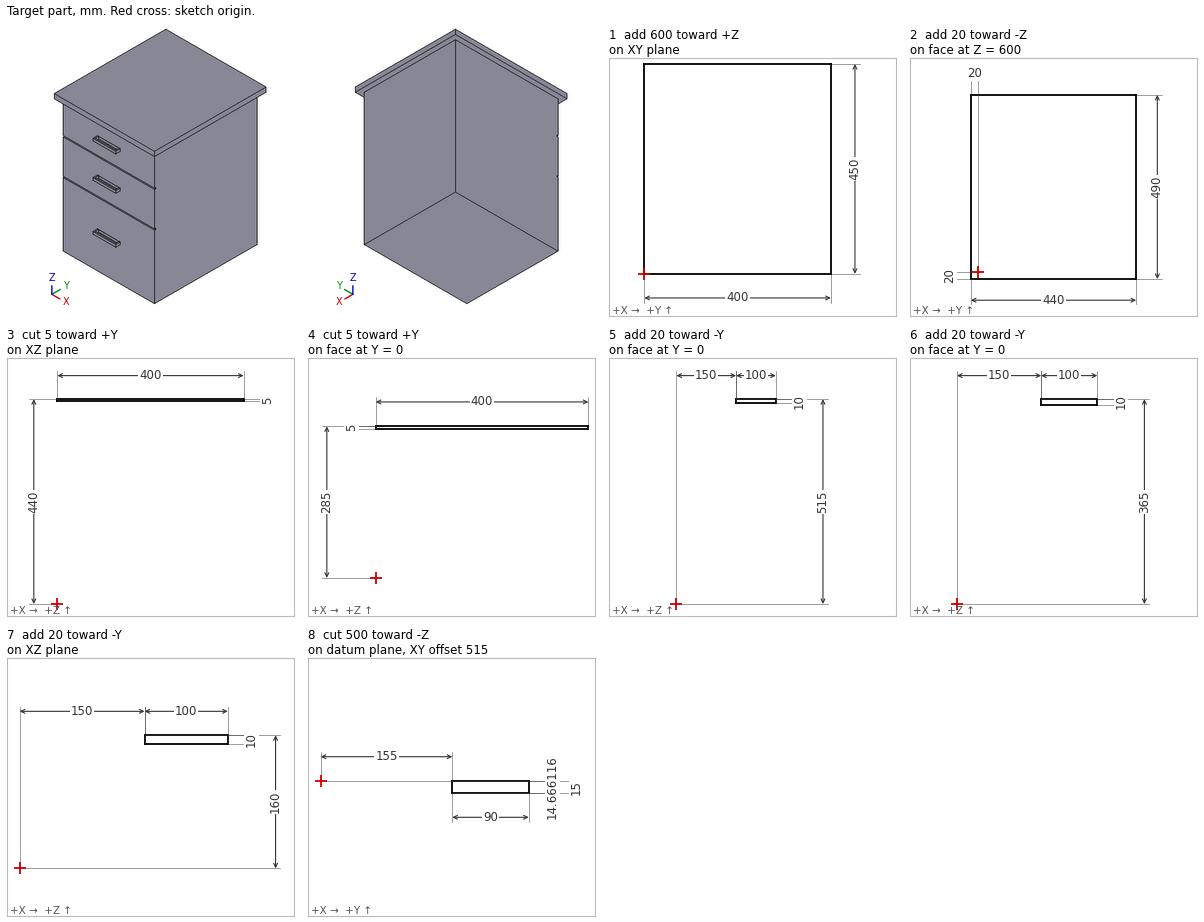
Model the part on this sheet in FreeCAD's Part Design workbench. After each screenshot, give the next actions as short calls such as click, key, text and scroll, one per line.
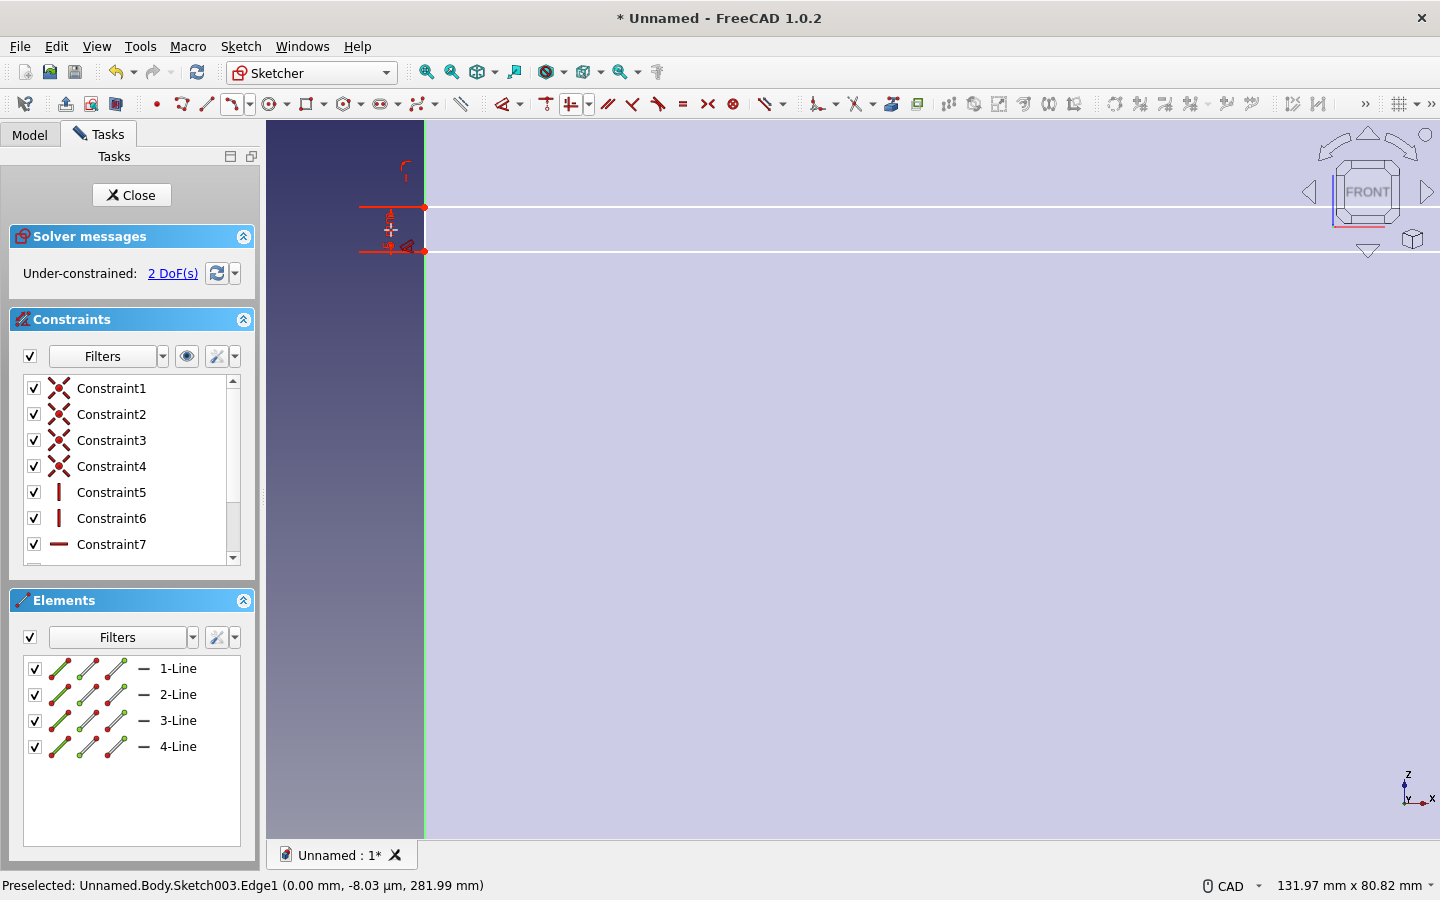
scroll(425, 228, down, 8)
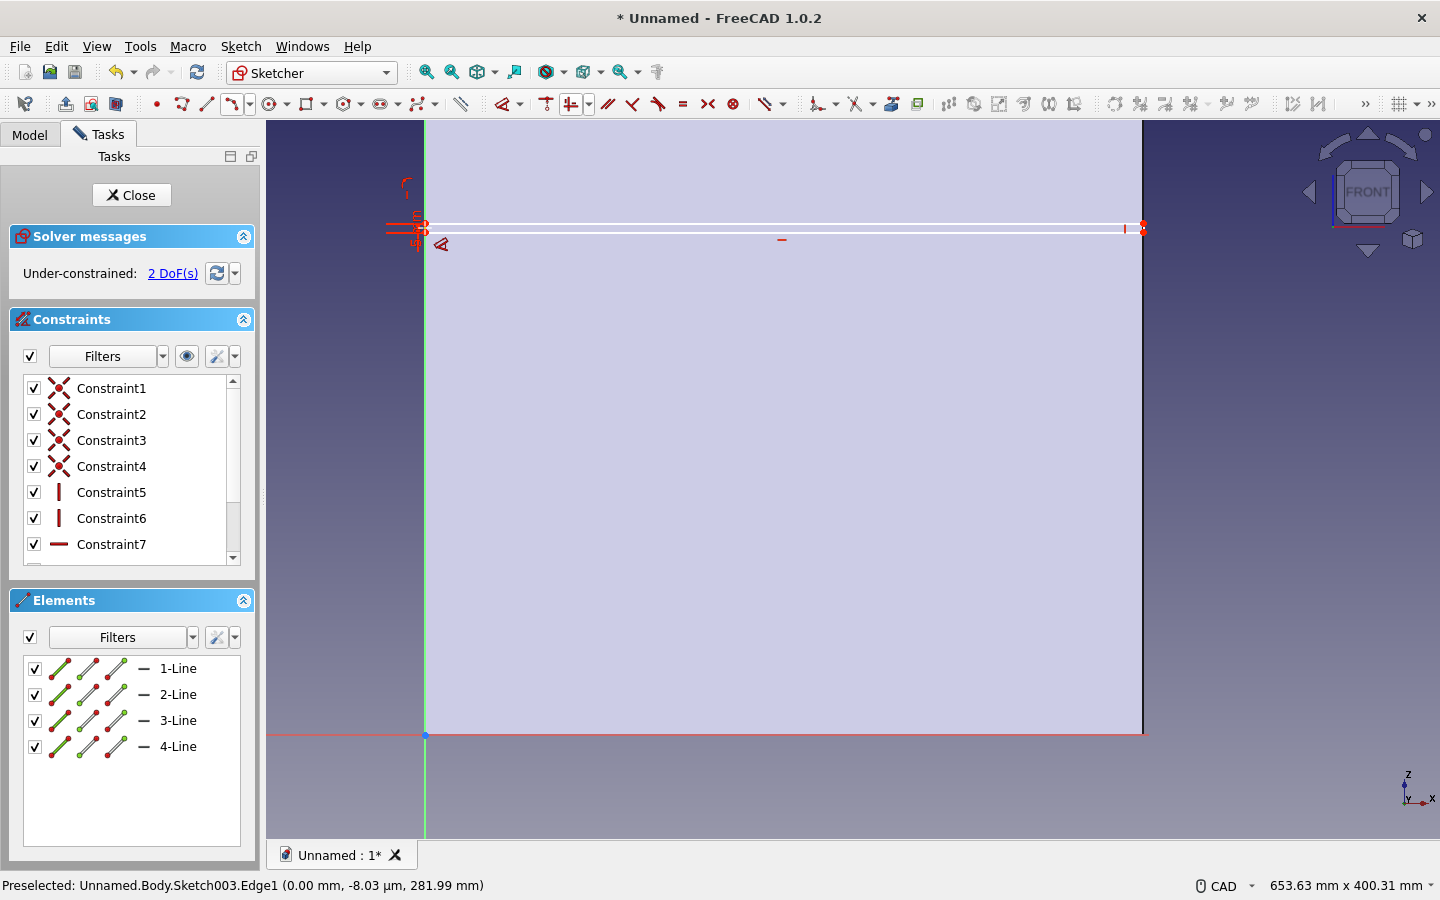
scroll(569, 233, up, 3)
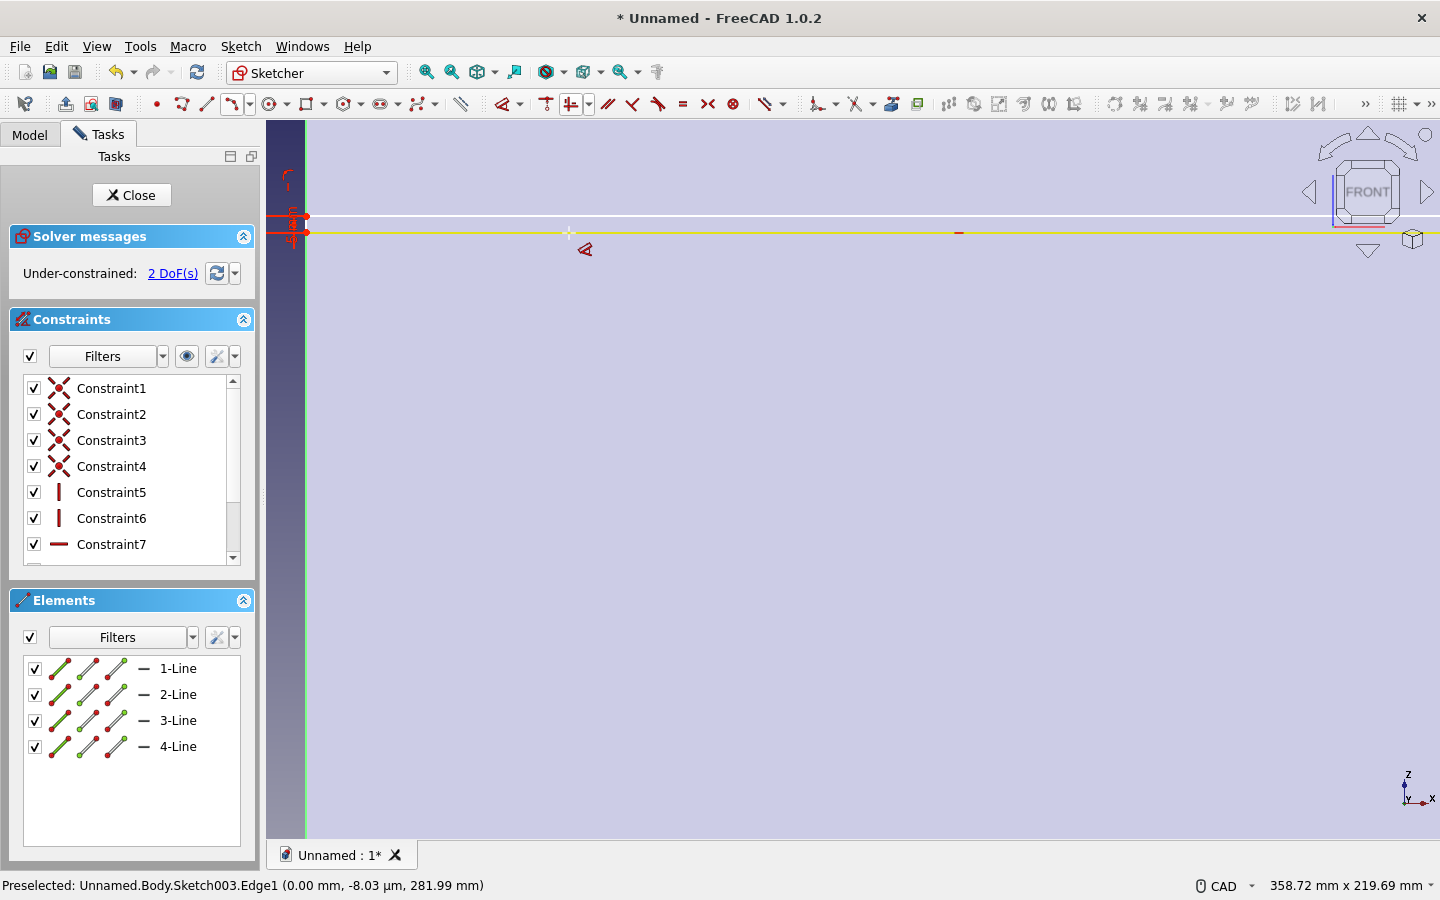
click(568, 233)
click(791, 199)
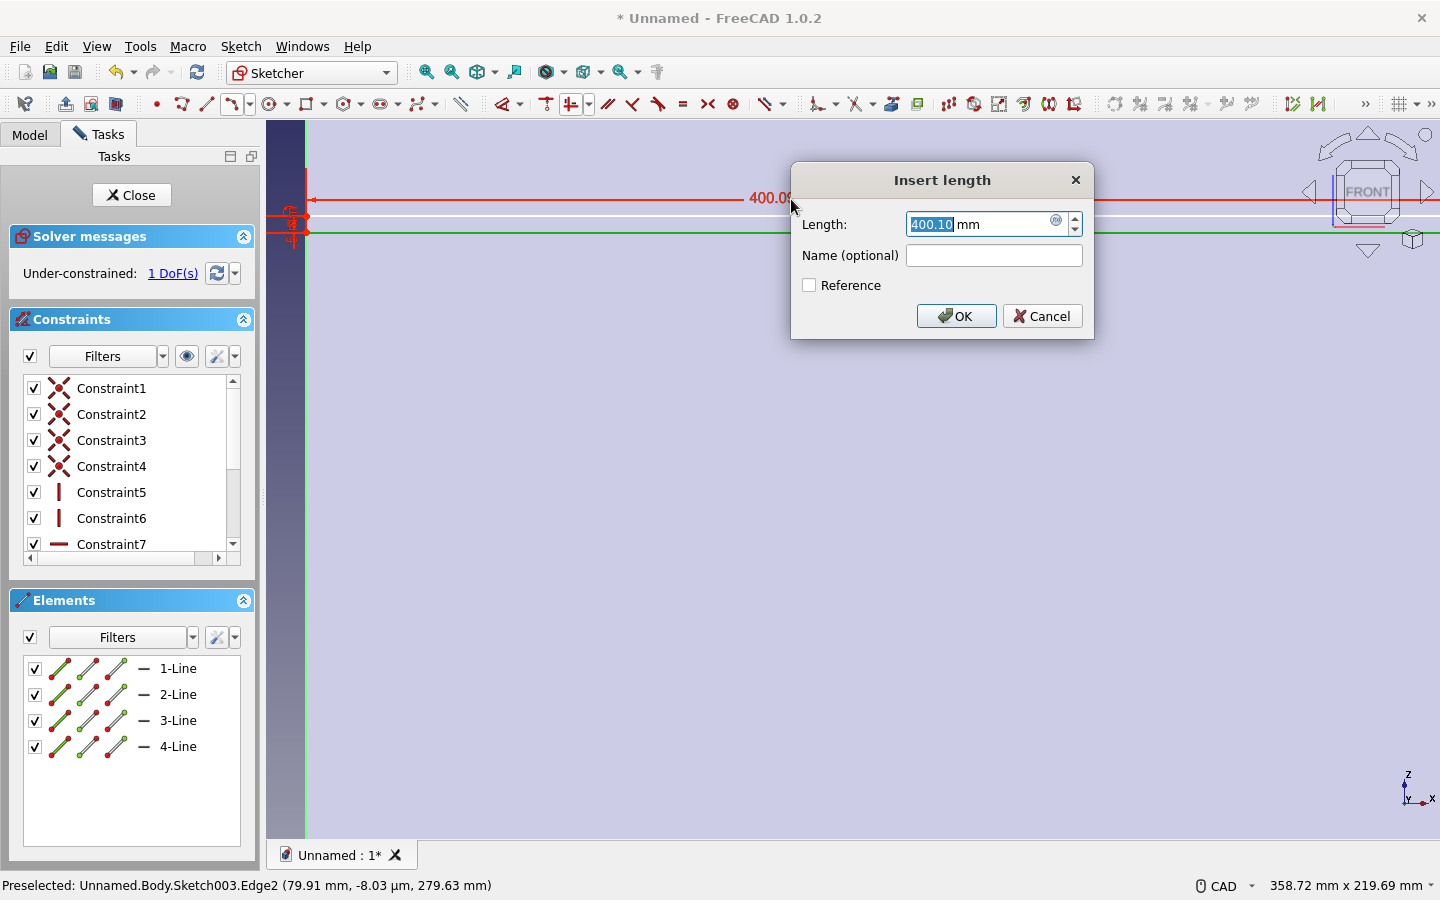
text(400)
key(Return)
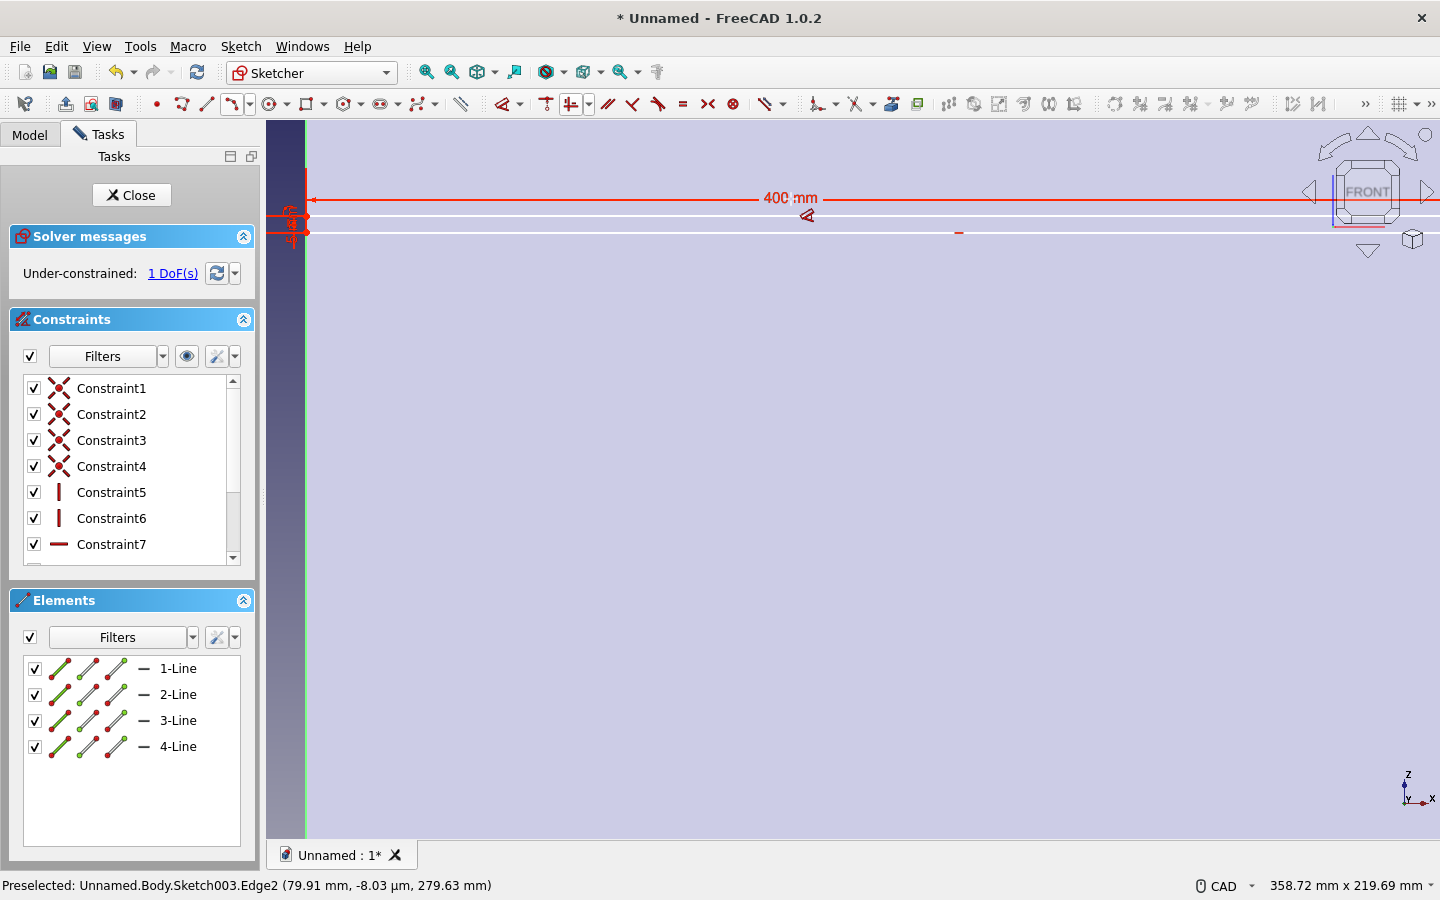
click(306, 216)
click(340, 514)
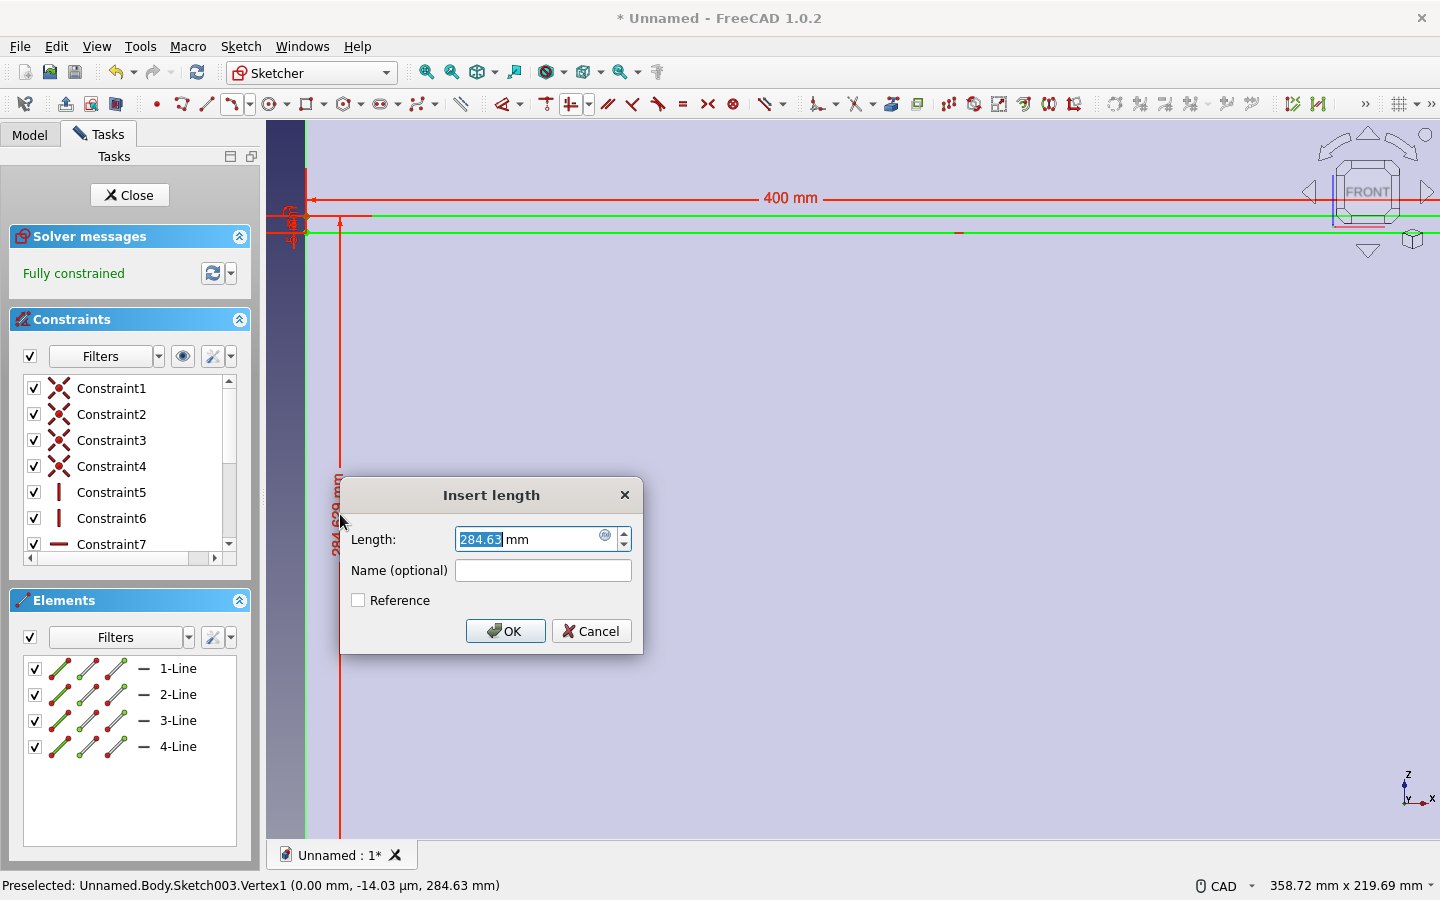
text(285)
key(Return)
key(Escape)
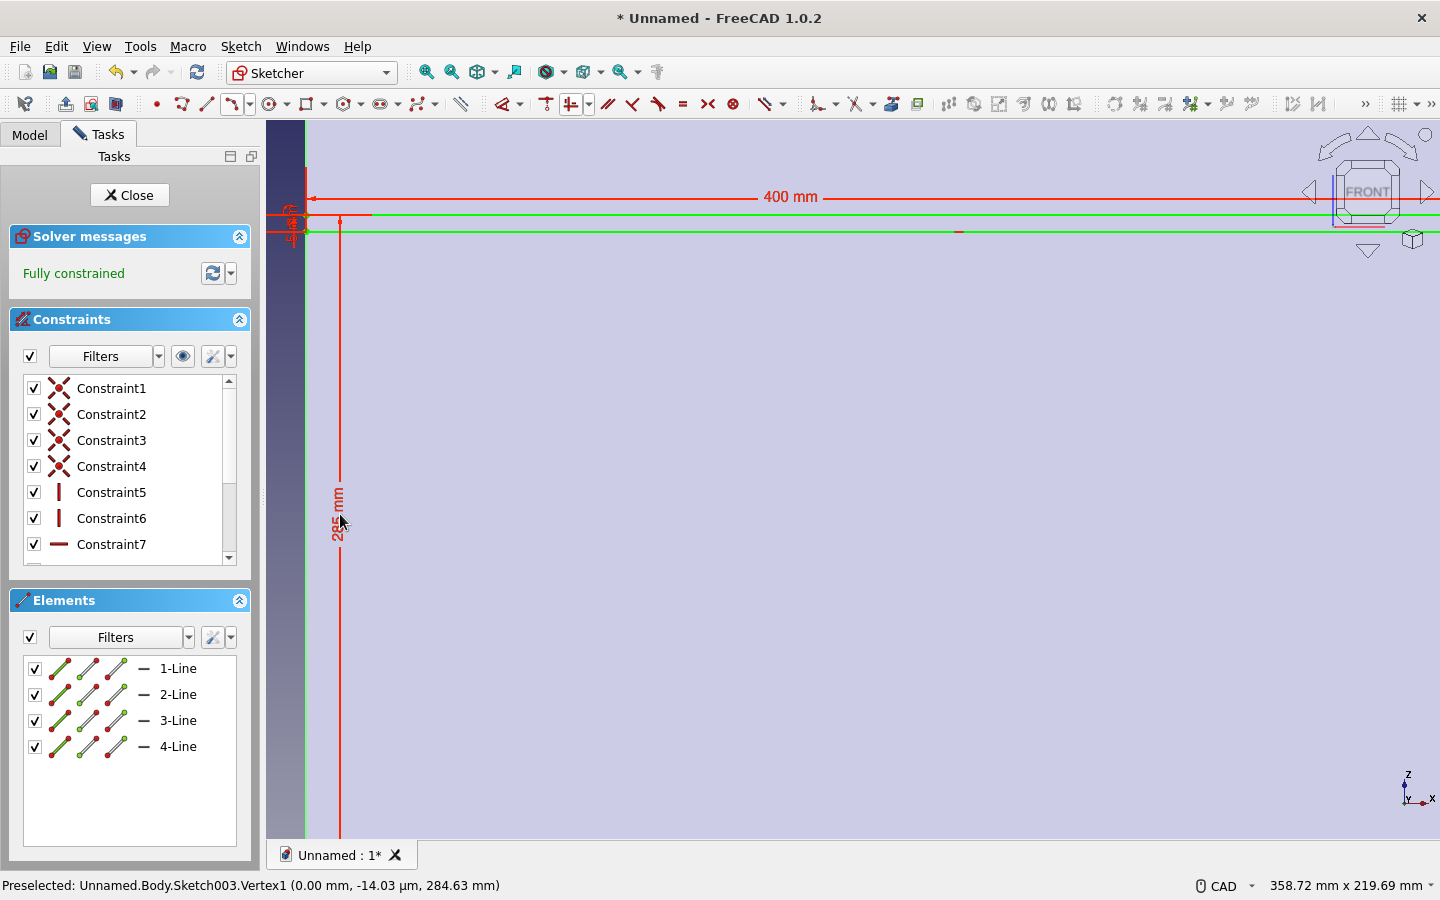
click(130, 195)